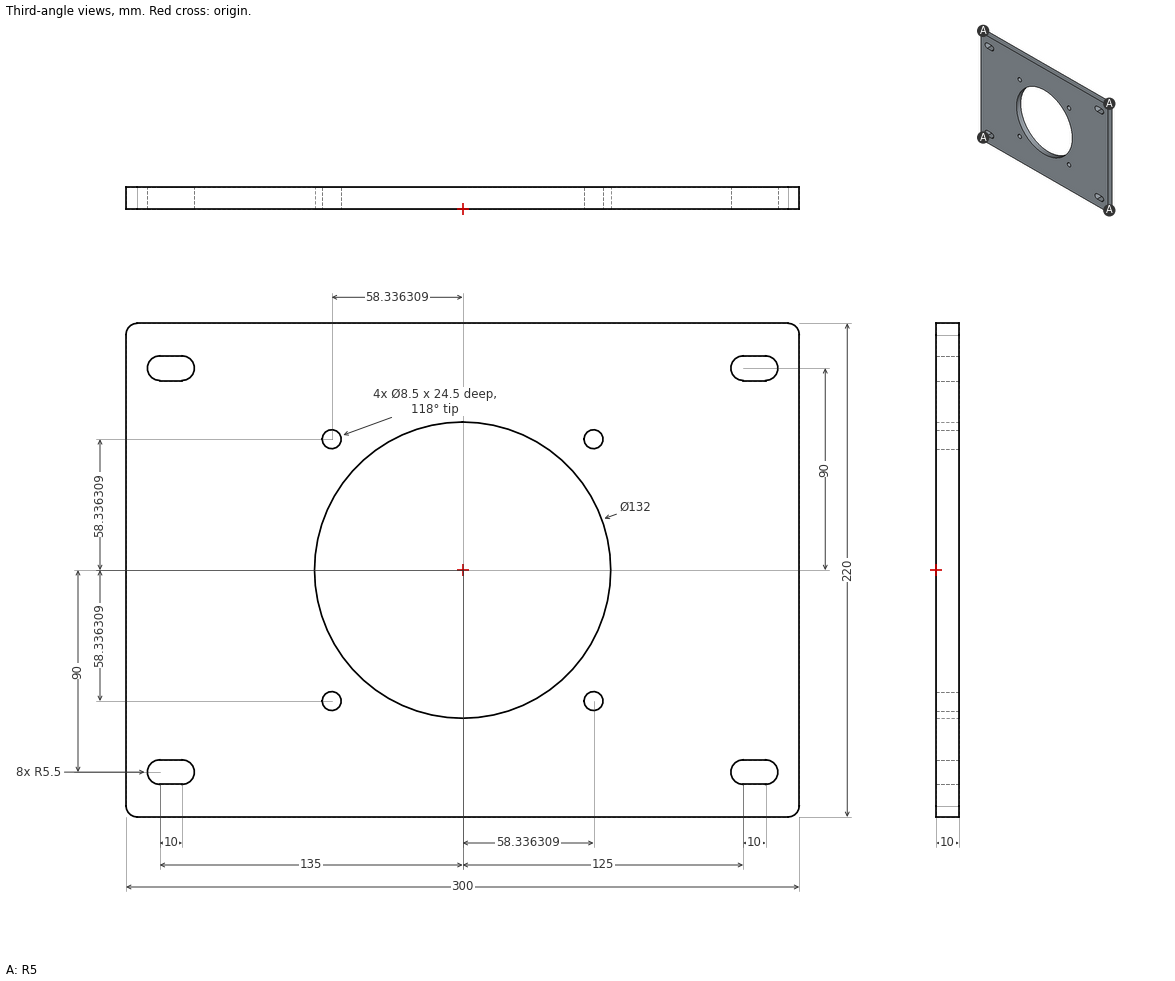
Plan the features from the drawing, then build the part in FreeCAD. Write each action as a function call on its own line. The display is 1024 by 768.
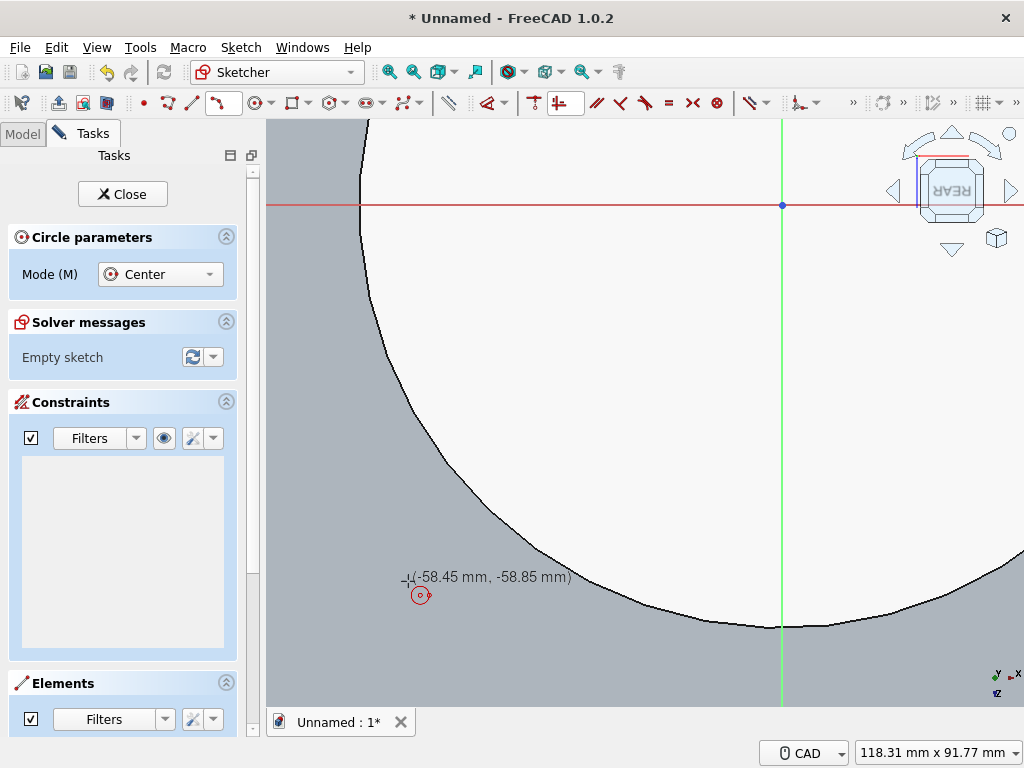
click(408, 579)
click(428, 560)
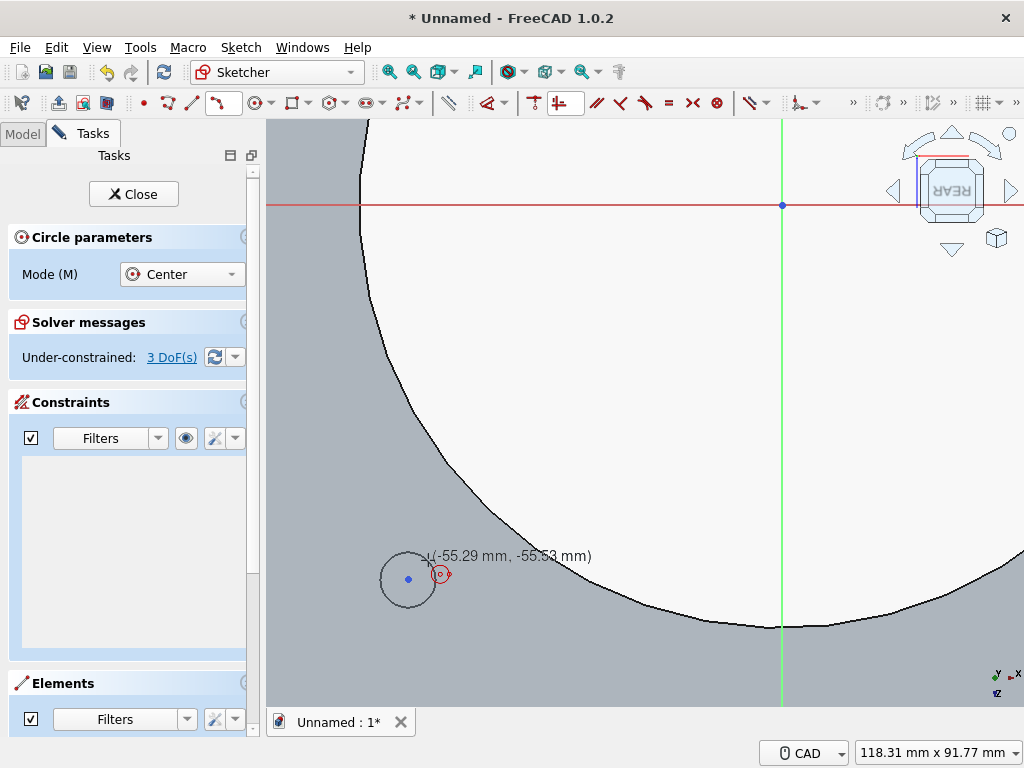
scroll(409, 583, down, 4)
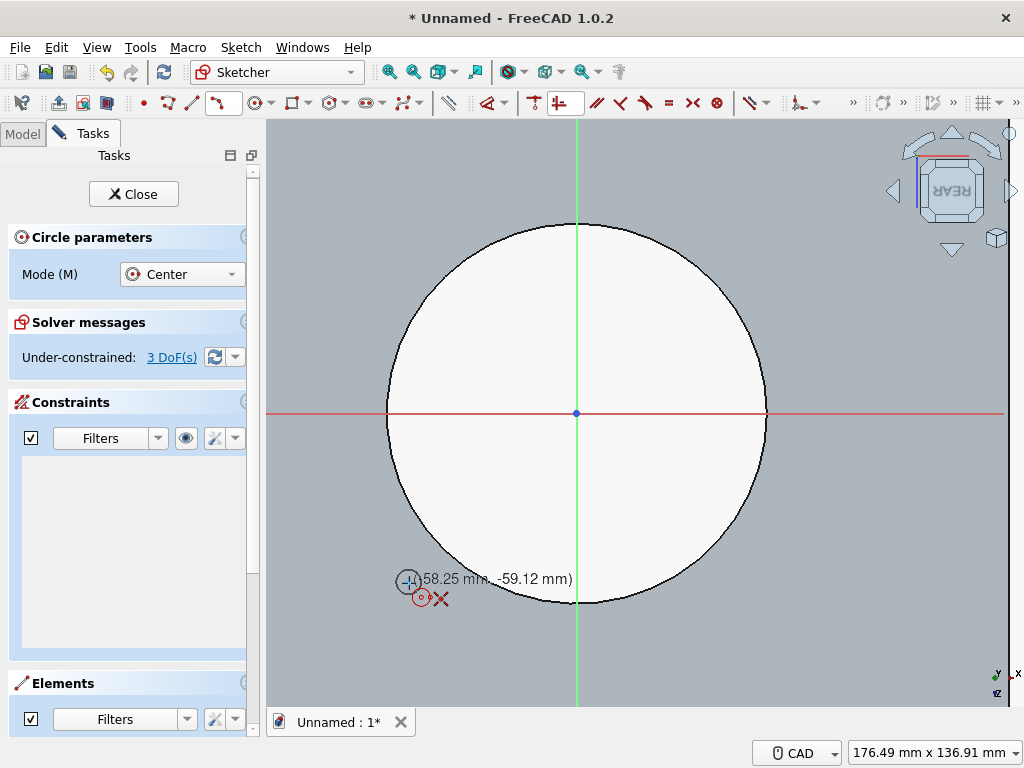
scroll(409, 246, up, 4)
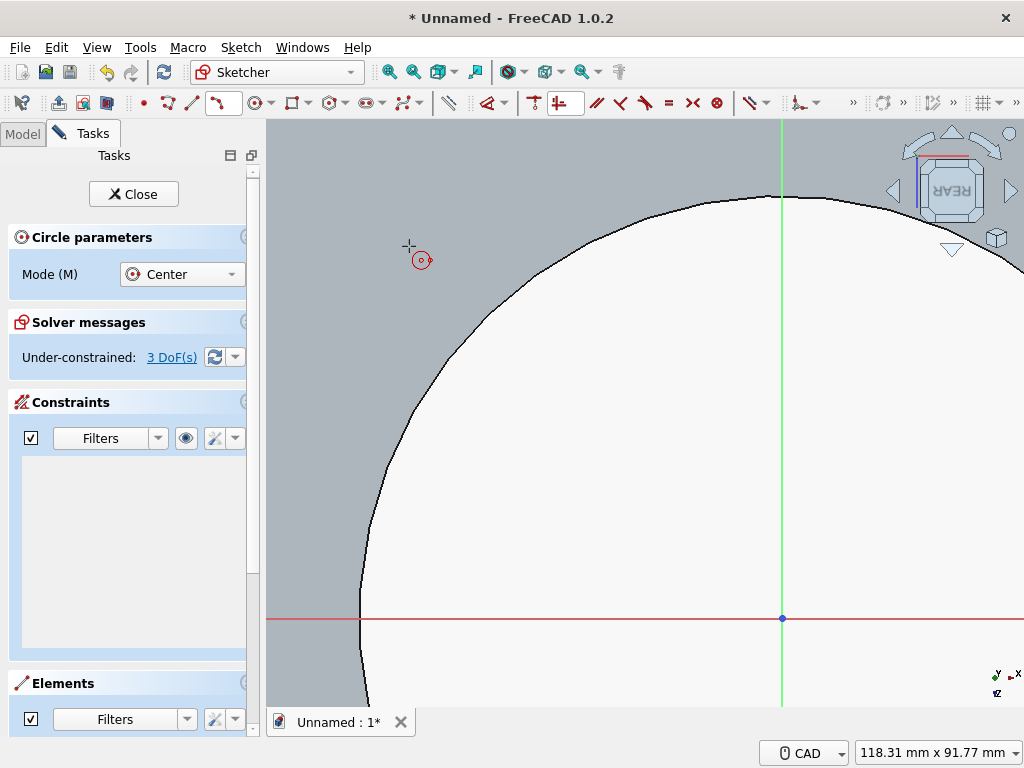
click(408, 245)
click(428, 226)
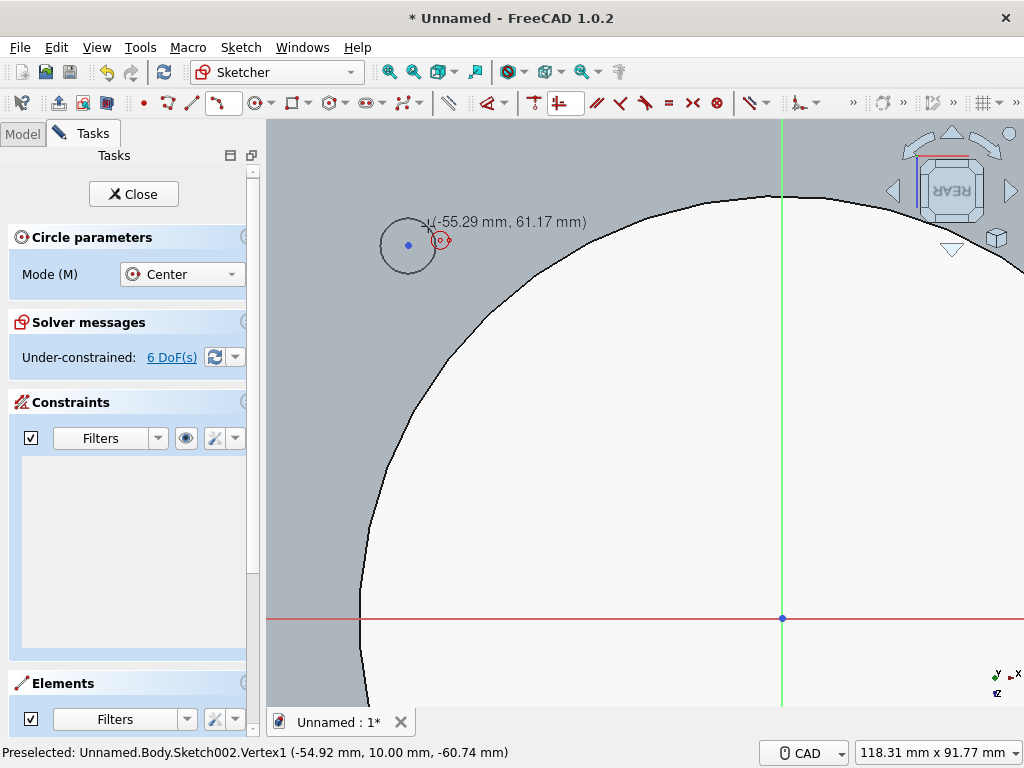
scroll(409, 245, down, 4)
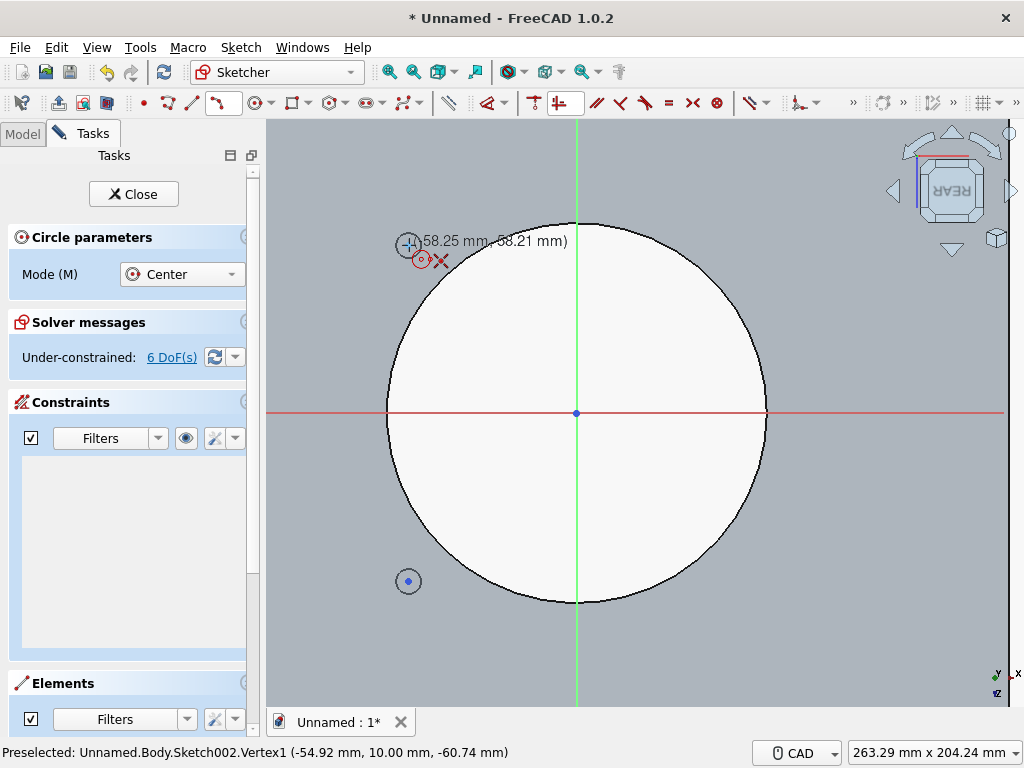
scroll(745, 245, up, 4)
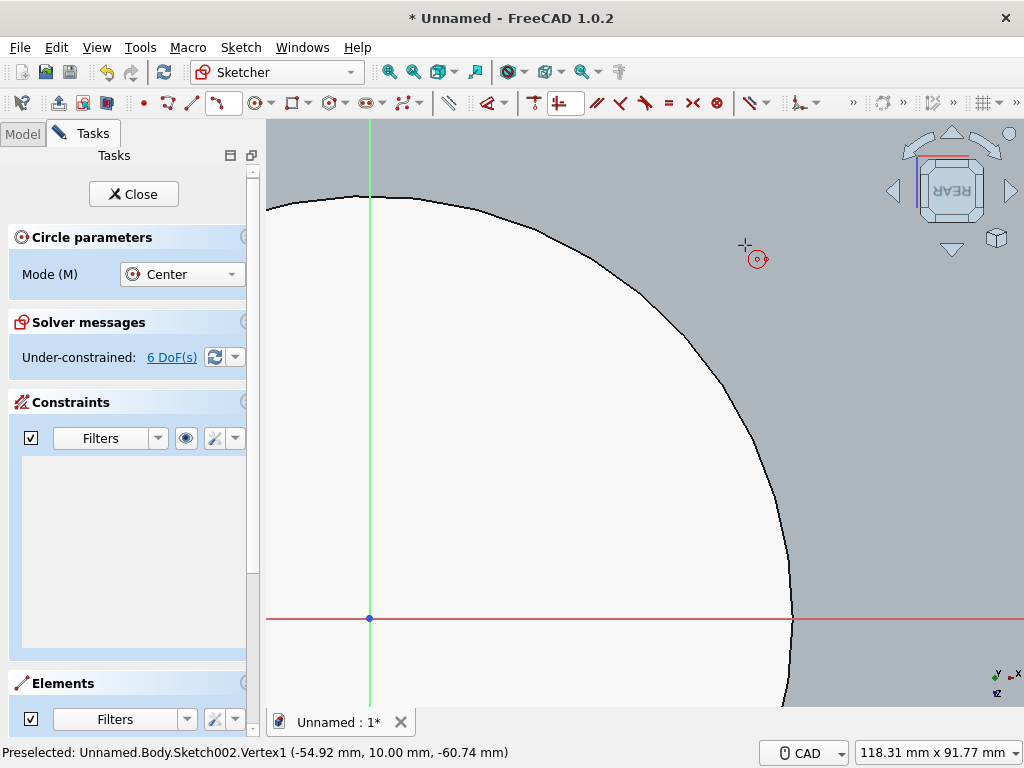
click(744, 245)
click(763, 226)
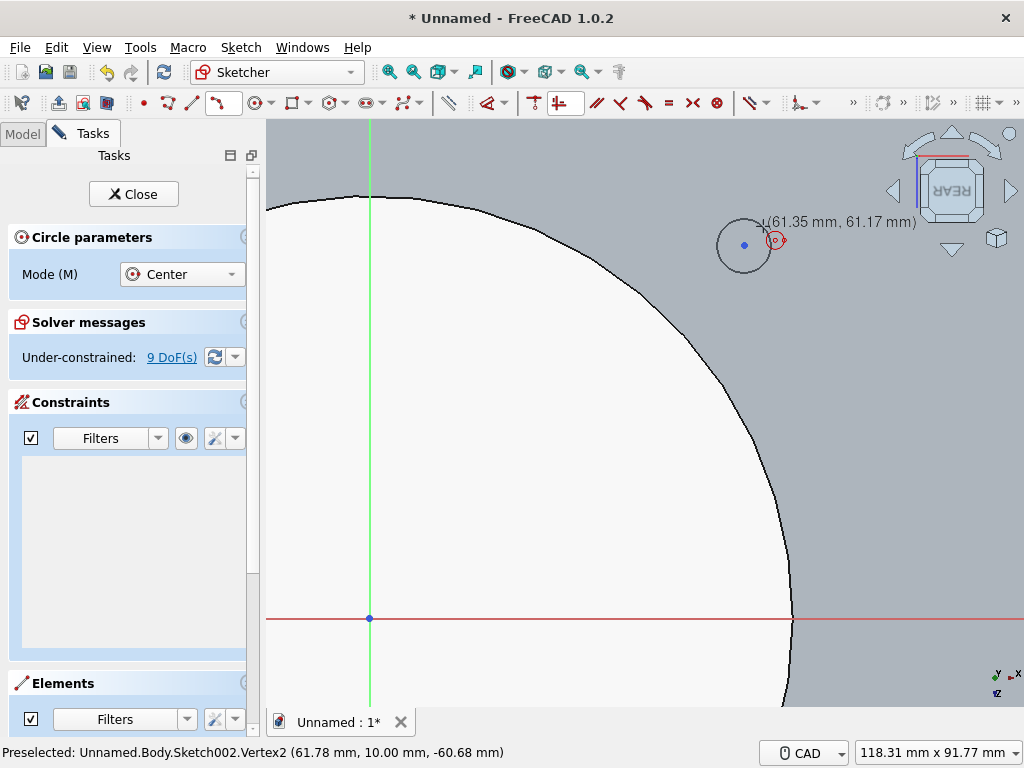
scroll(745, 245, down, 4)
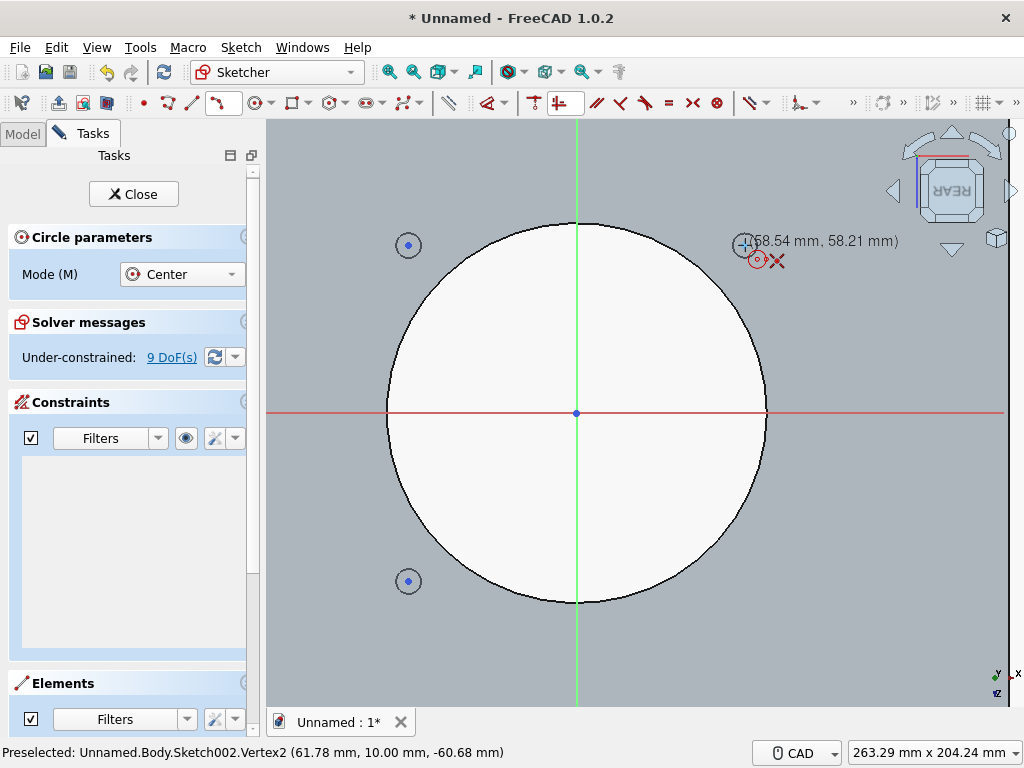
scroll(745, 581, up, 4)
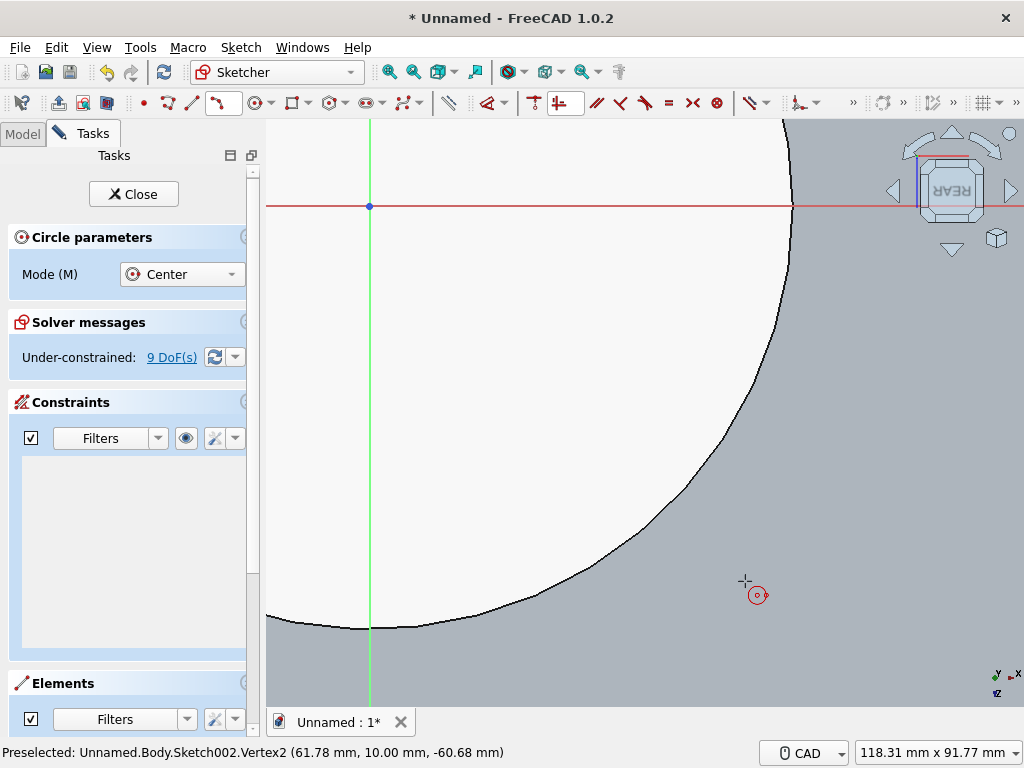
click(744, 580)
click(763, 561)
key(Escape)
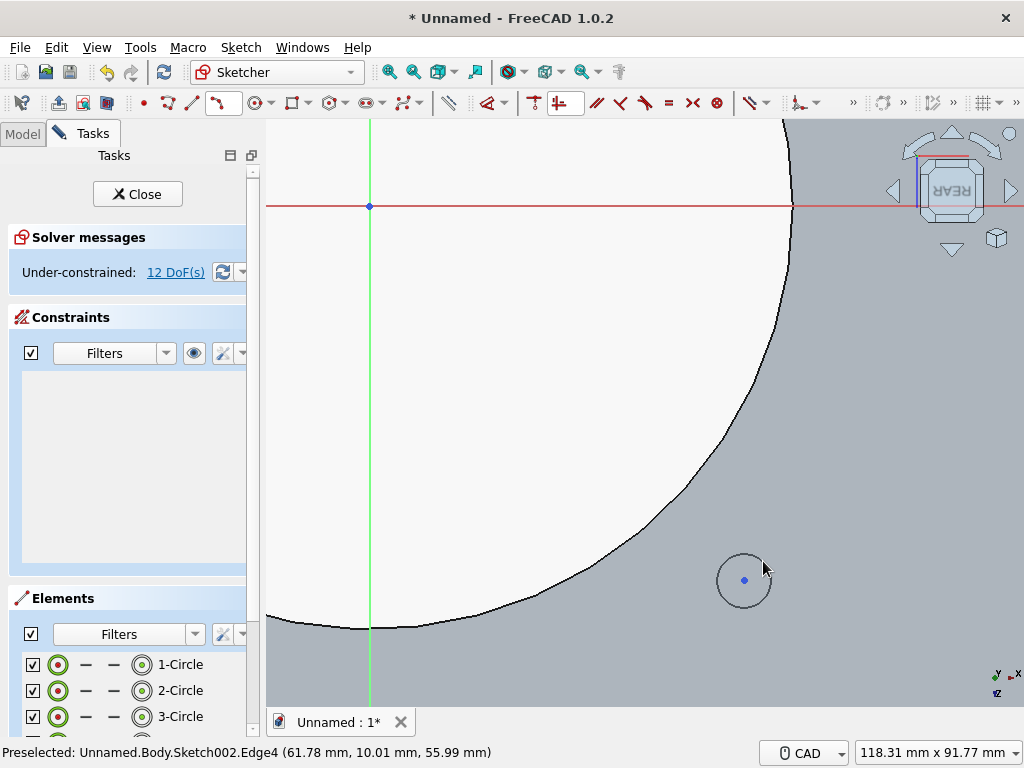
scroll(745, 582, down, 4)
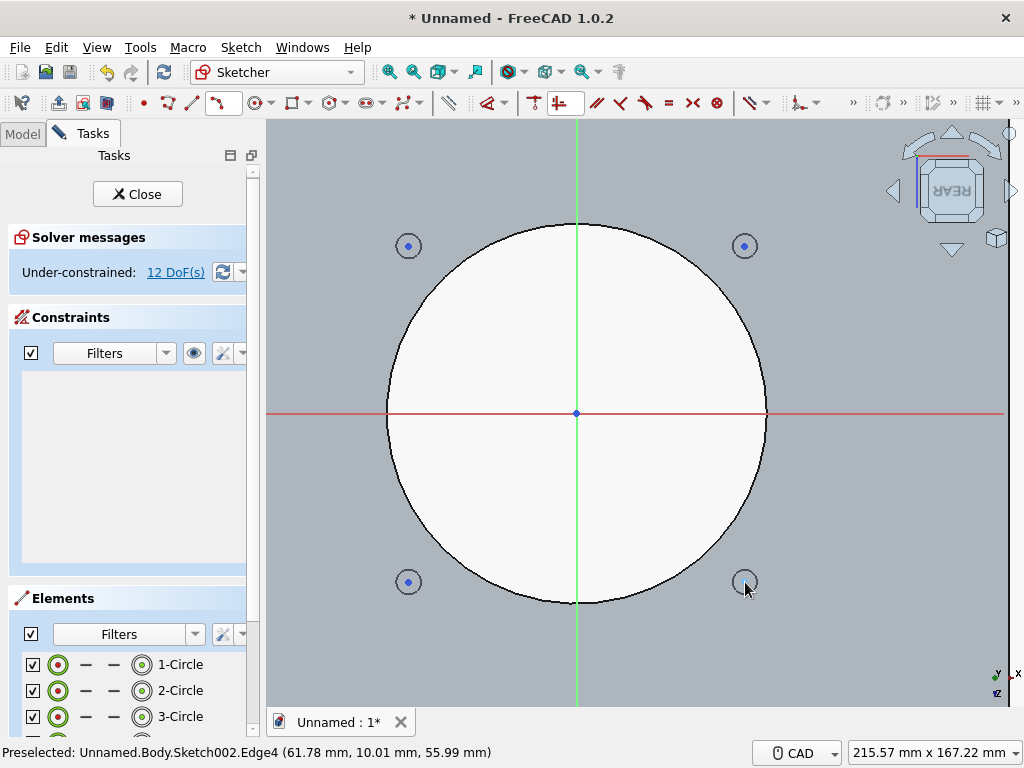
click(417, 573)